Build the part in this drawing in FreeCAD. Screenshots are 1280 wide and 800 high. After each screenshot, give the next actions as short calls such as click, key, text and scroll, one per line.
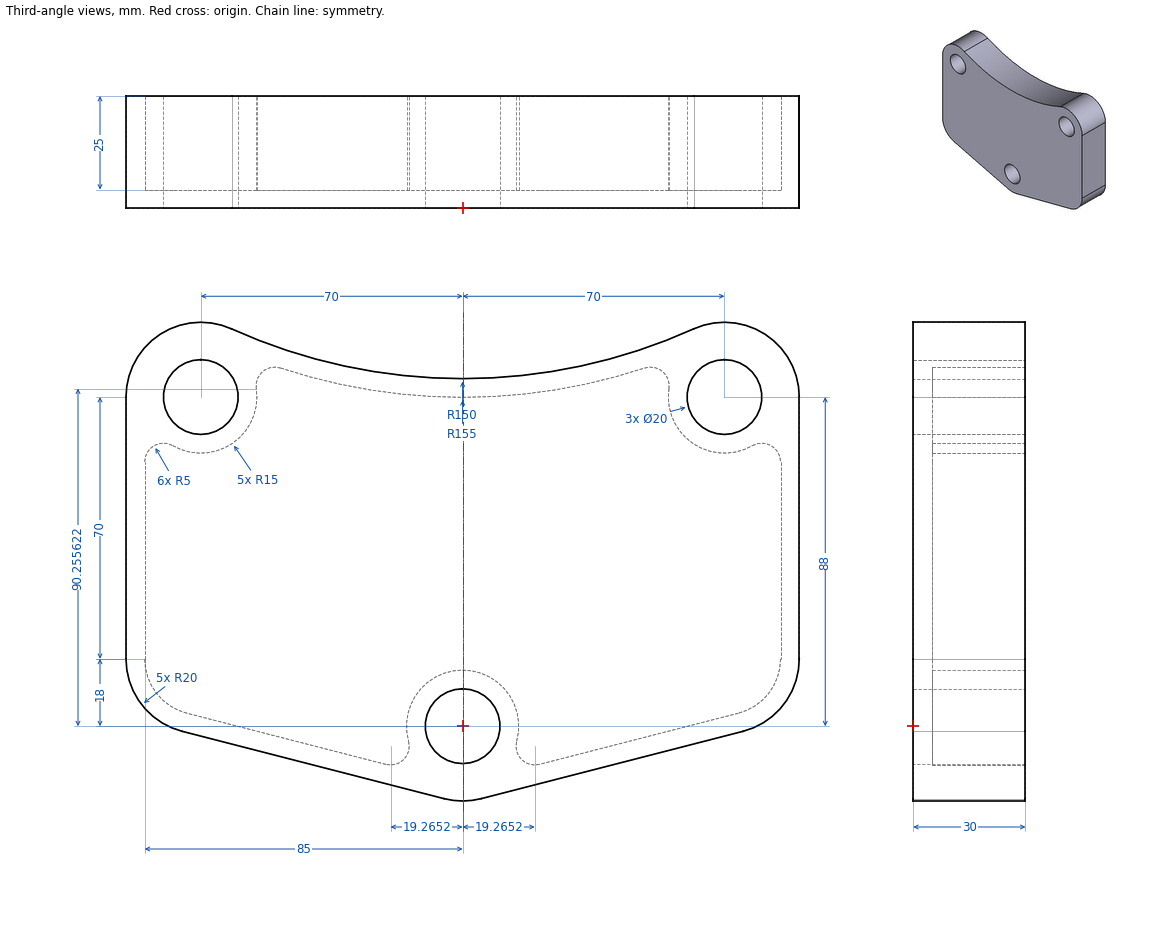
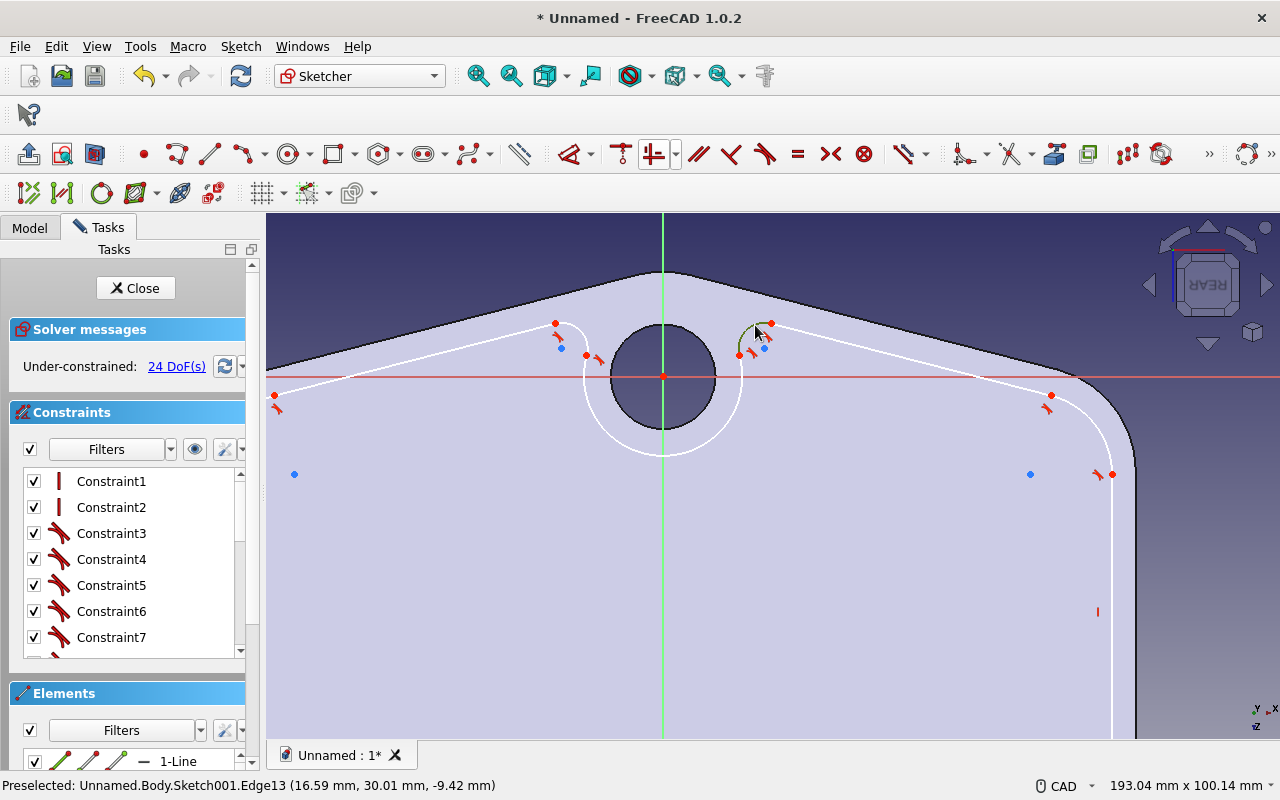
click(586, 340)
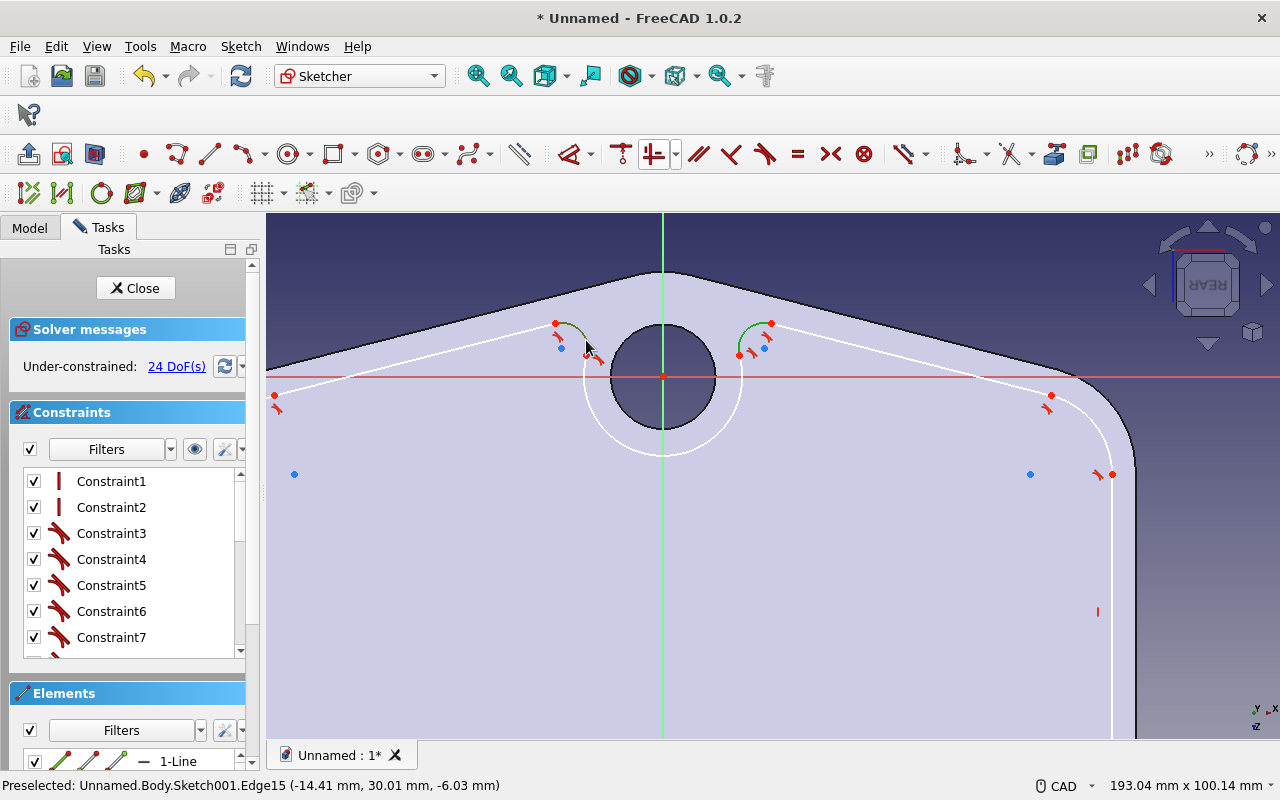
click(798, 154)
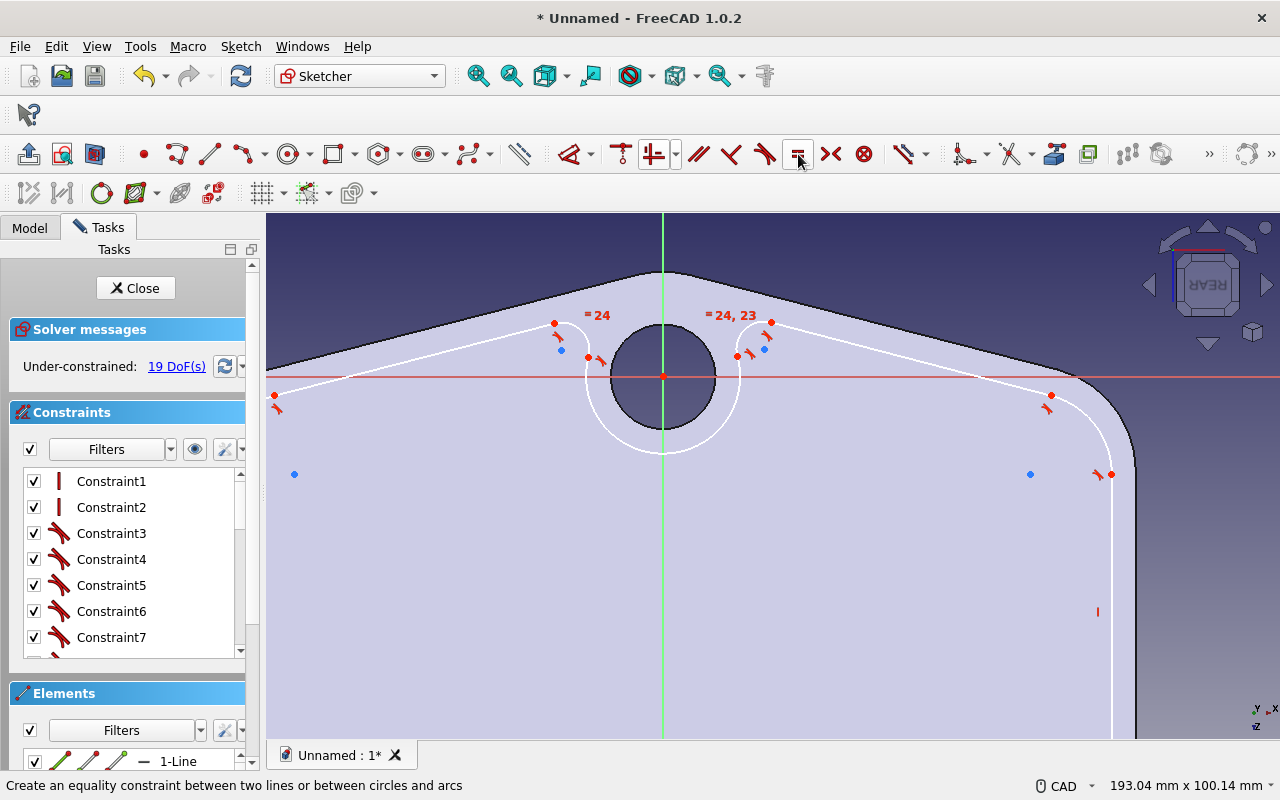
scroll(755, 324, down, 3)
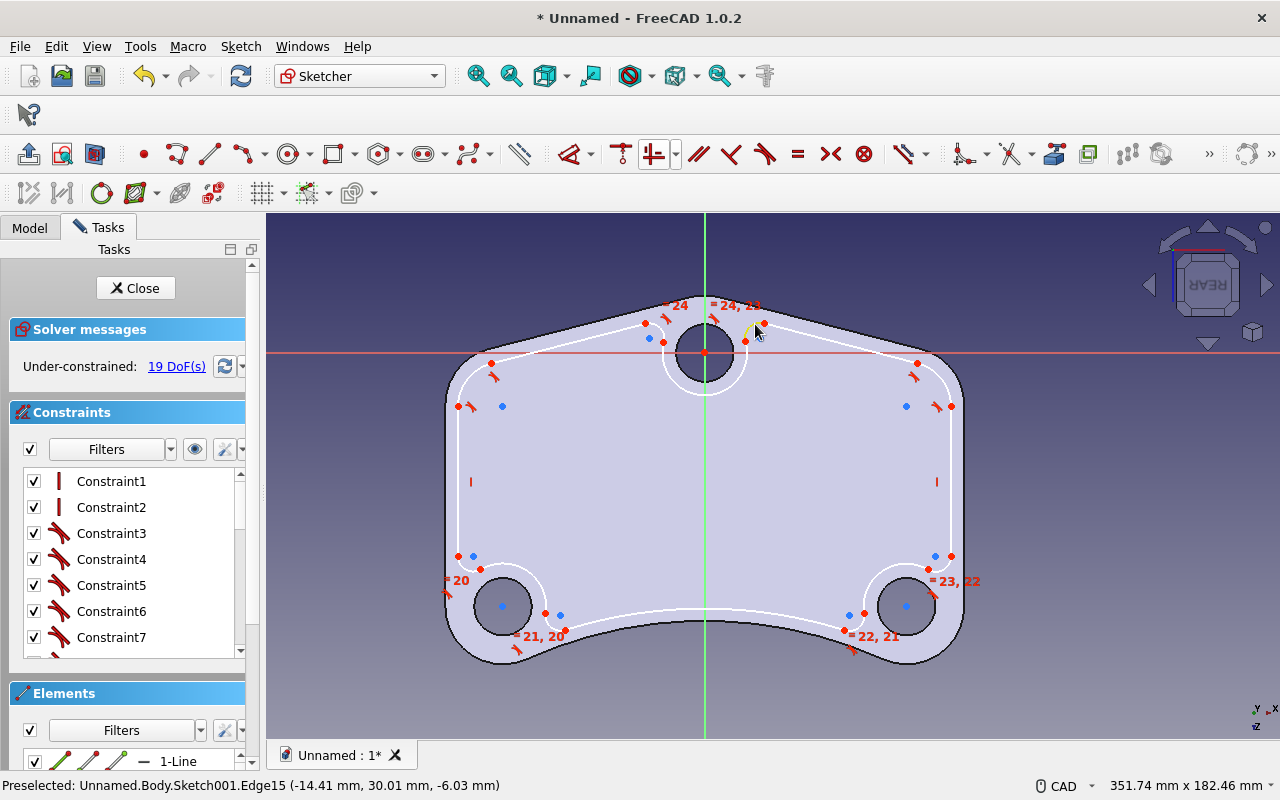
click(540, 585)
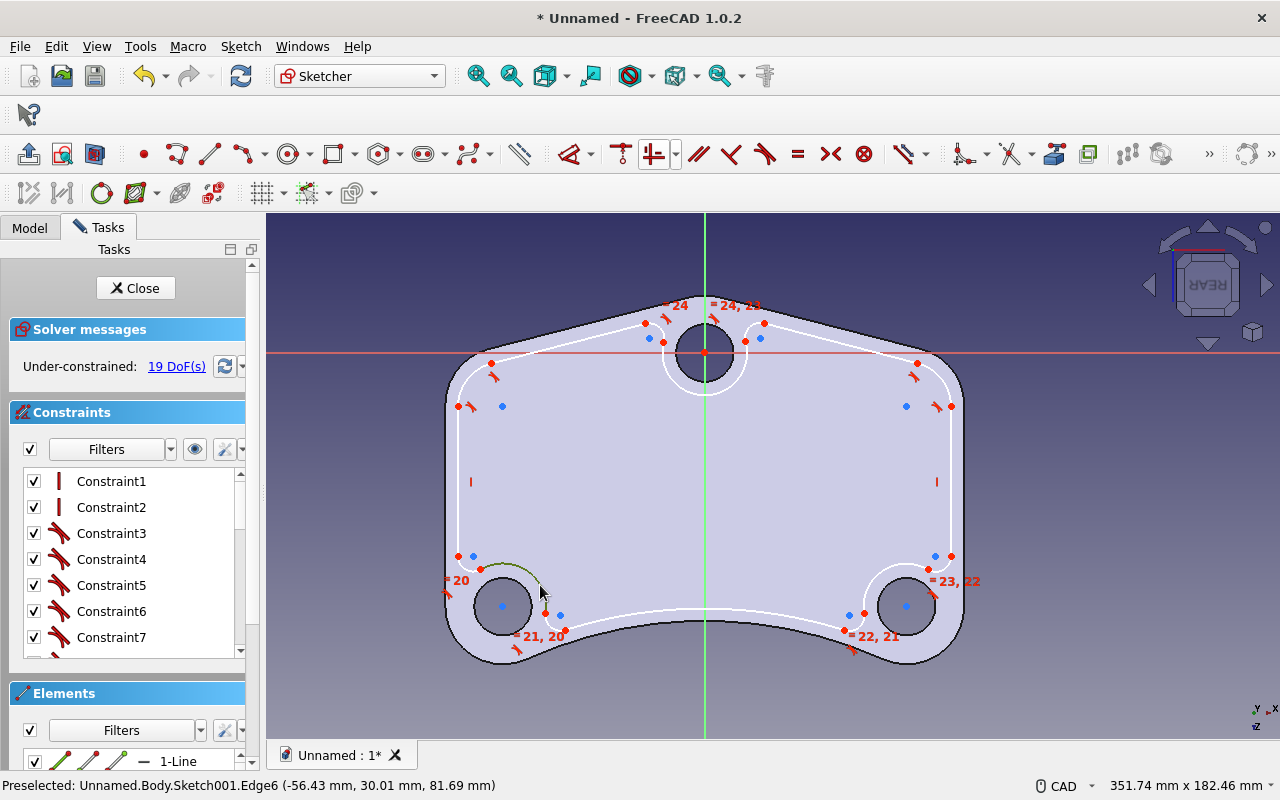
click(900, 564)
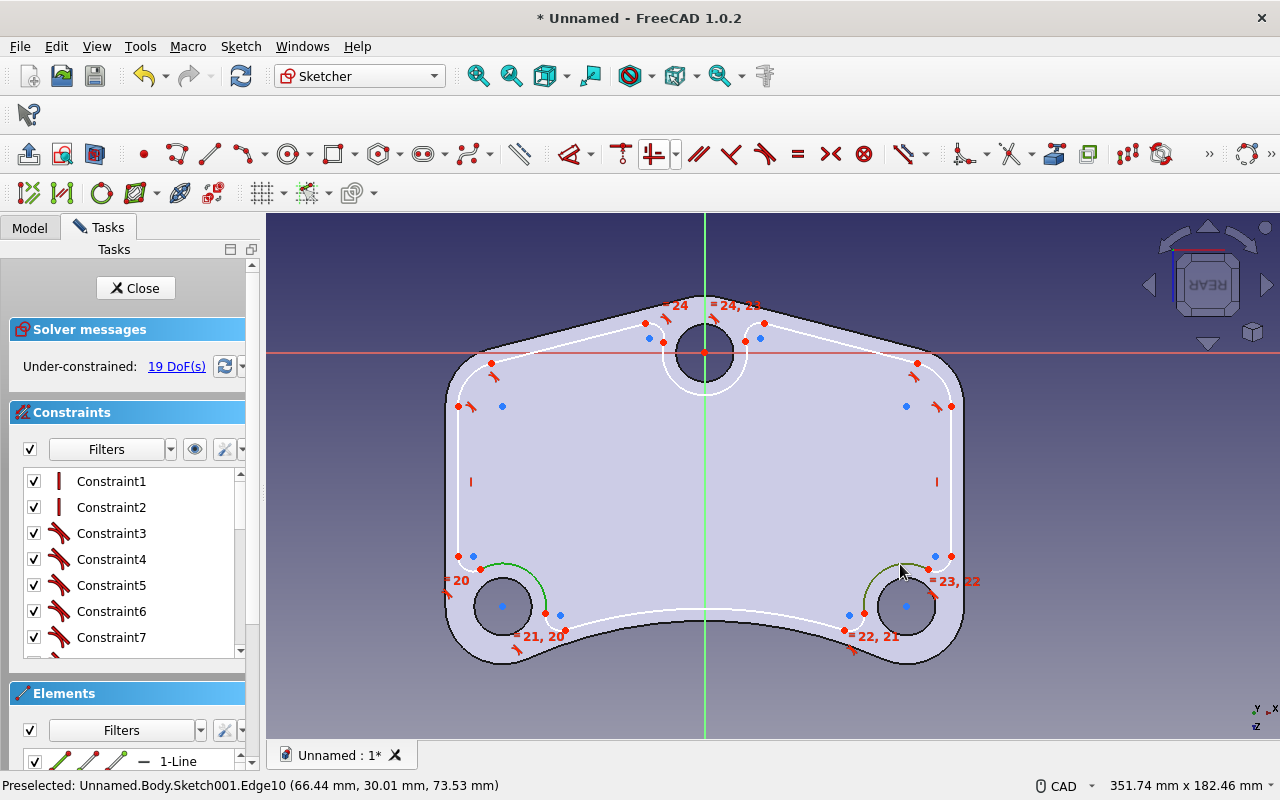
click(948, 389)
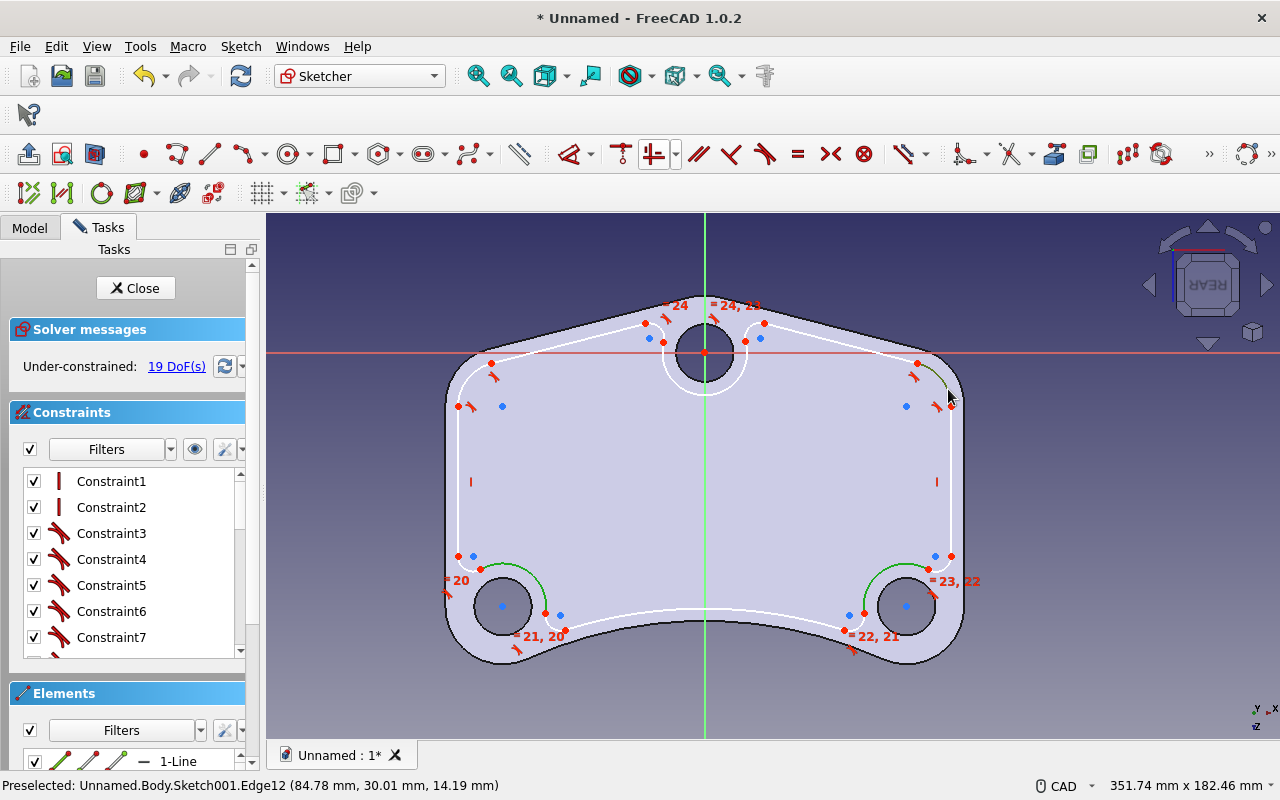
click(677, 385)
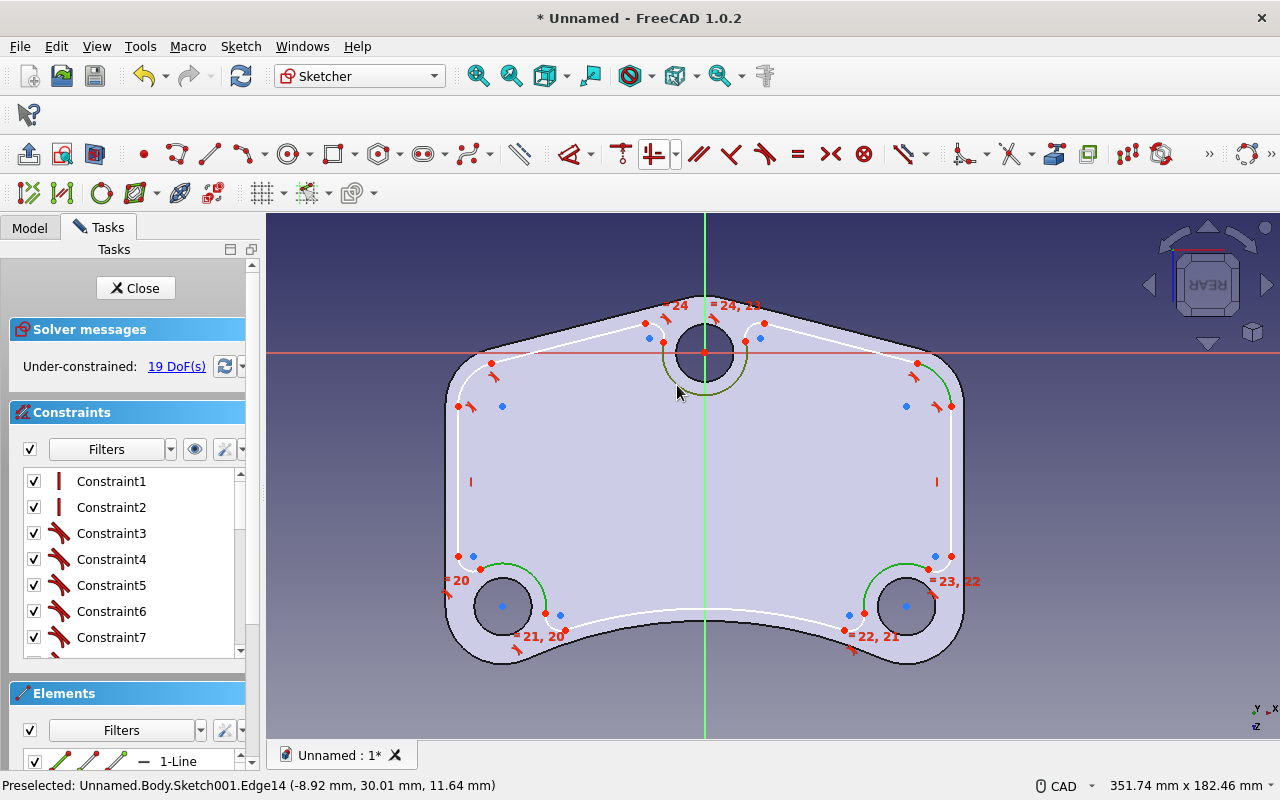
click(476, 371)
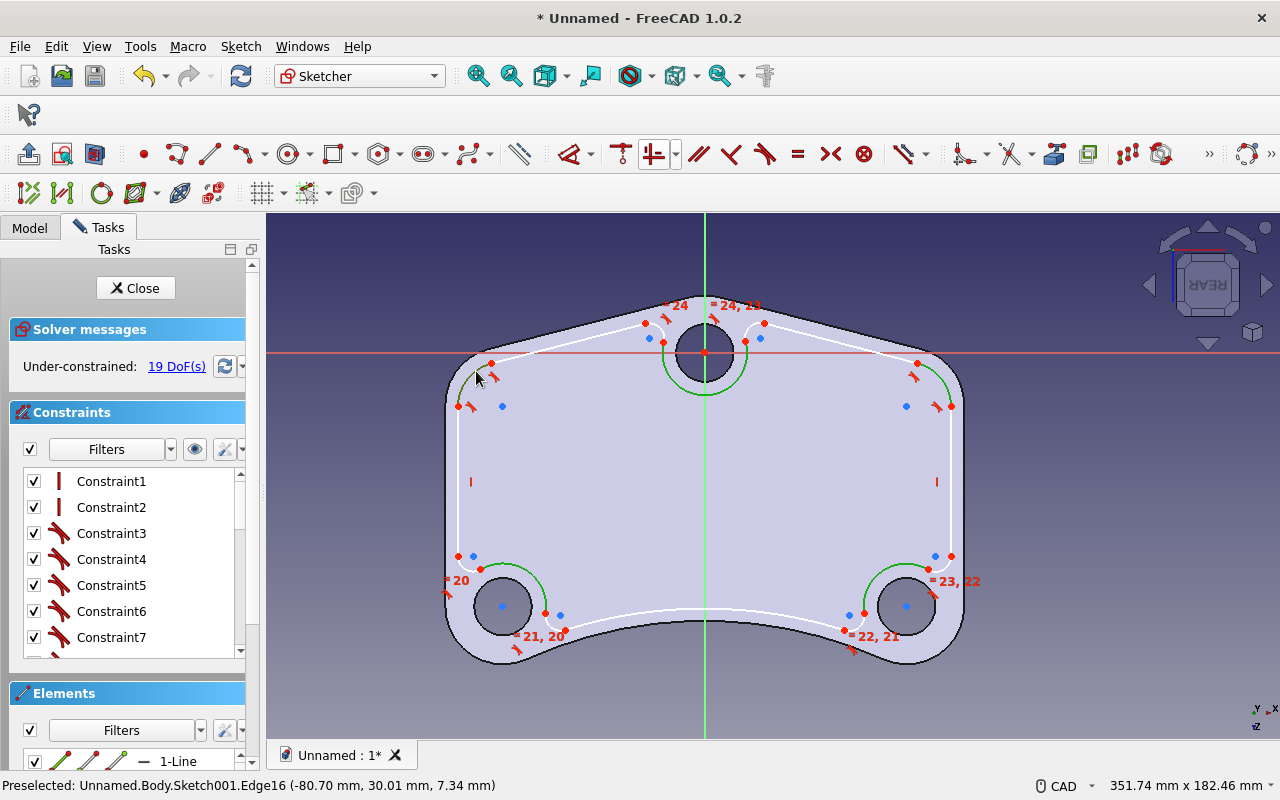
click(798, 154)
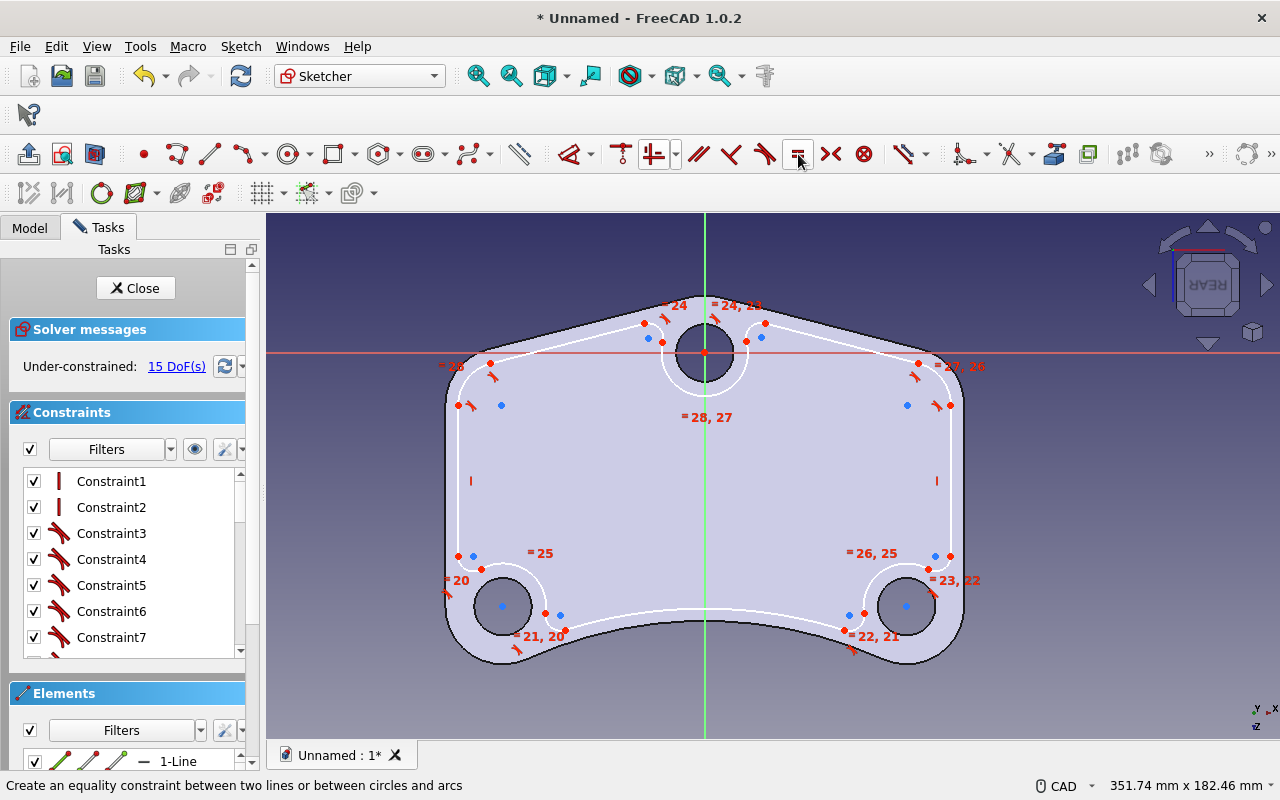
scroll(704, 295, down, 4)